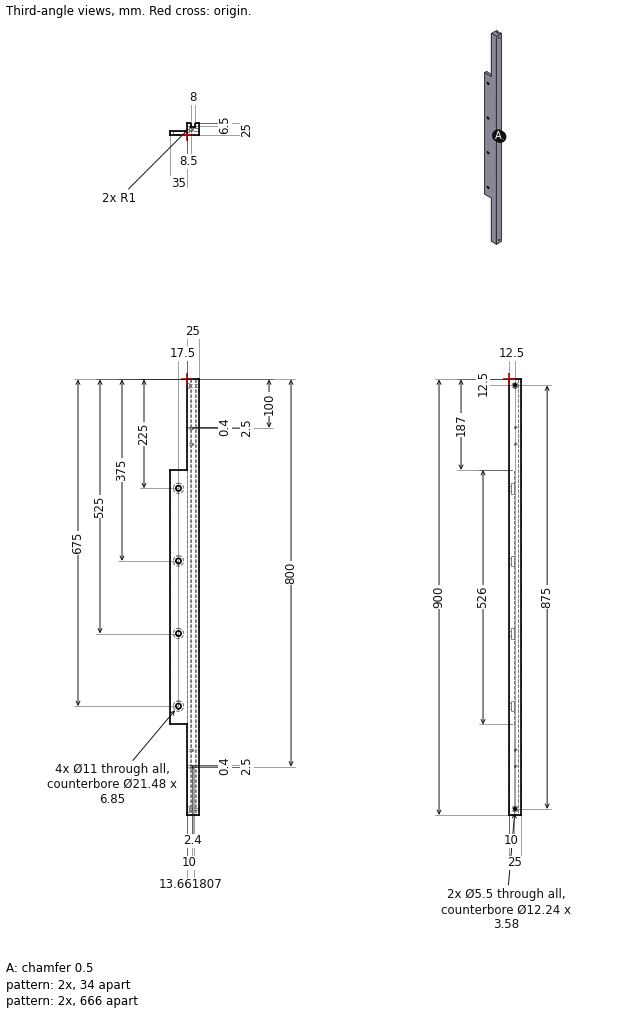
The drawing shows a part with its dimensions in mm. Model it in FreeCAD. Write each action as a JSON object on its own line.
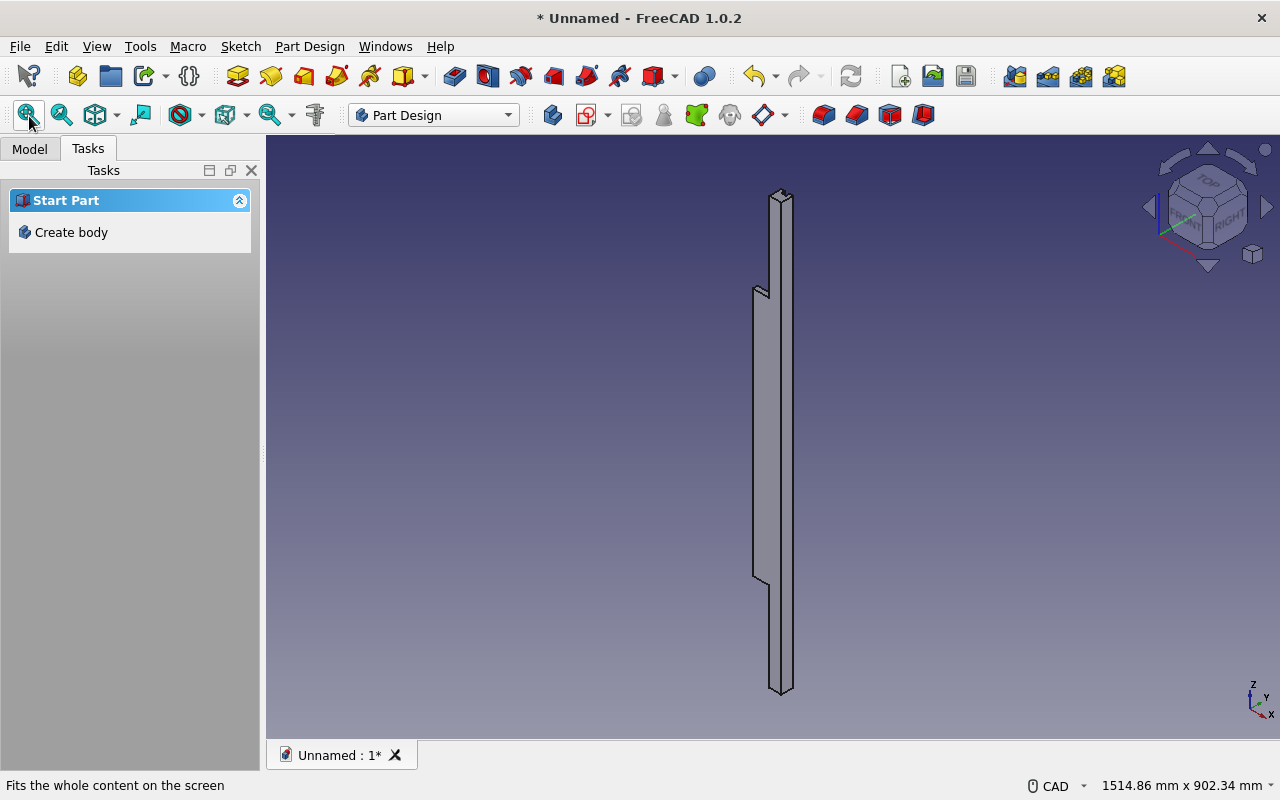
{"action": "key", "text": "2"}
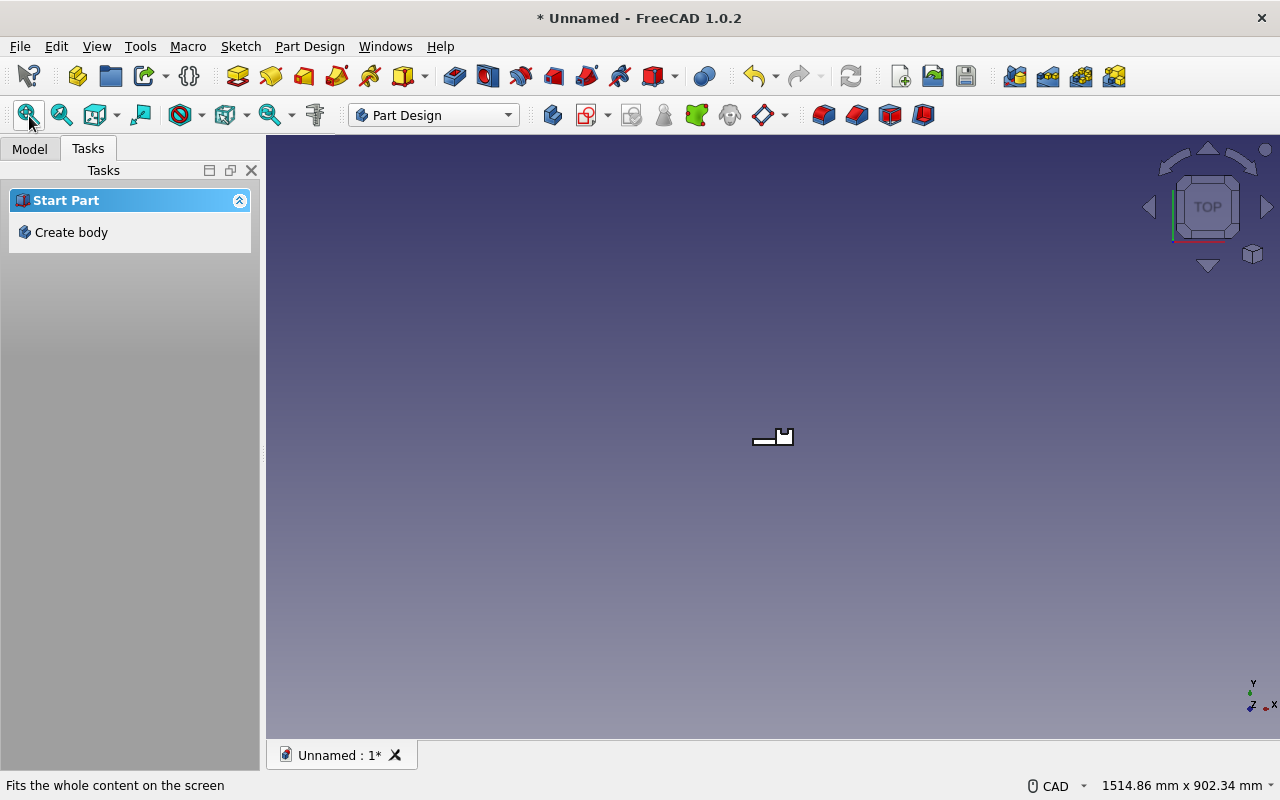
{"action": "left_click", "coordinate": [29, 116]}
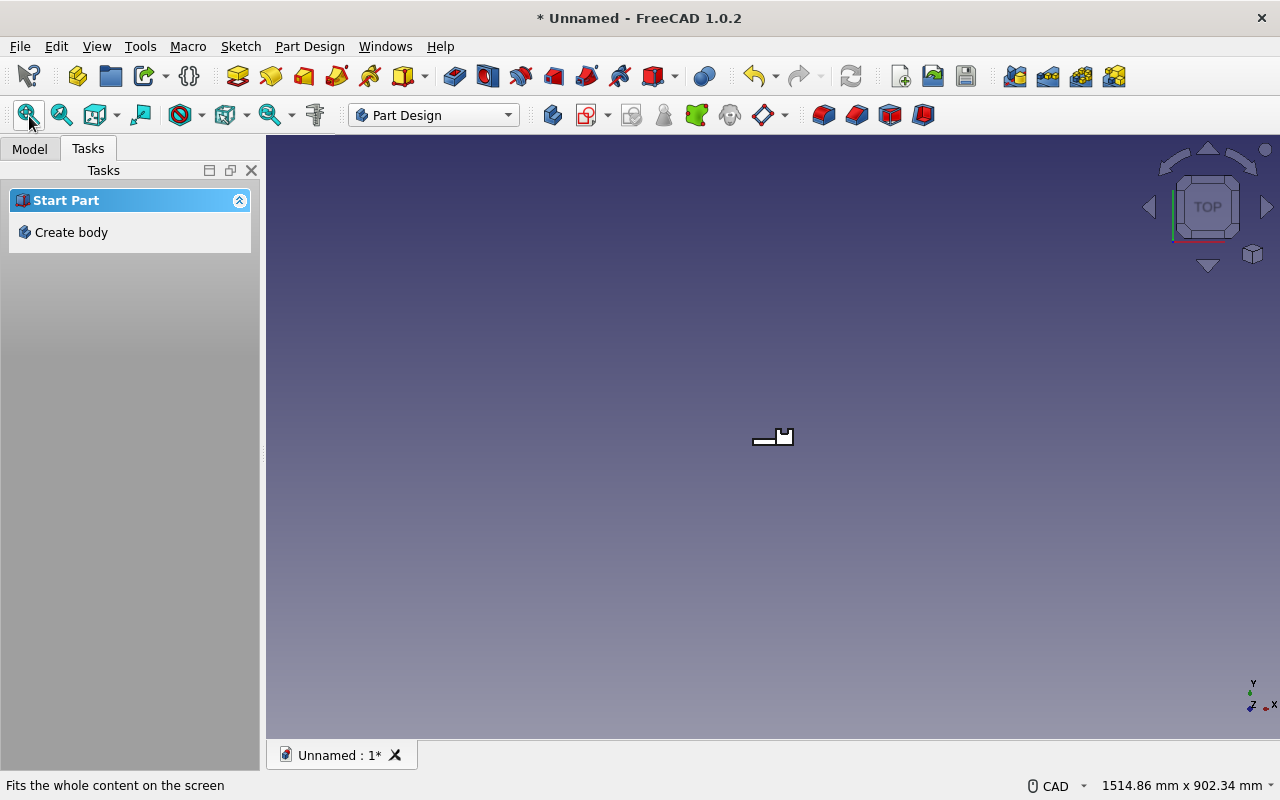
{"action": "key", "text": "1"}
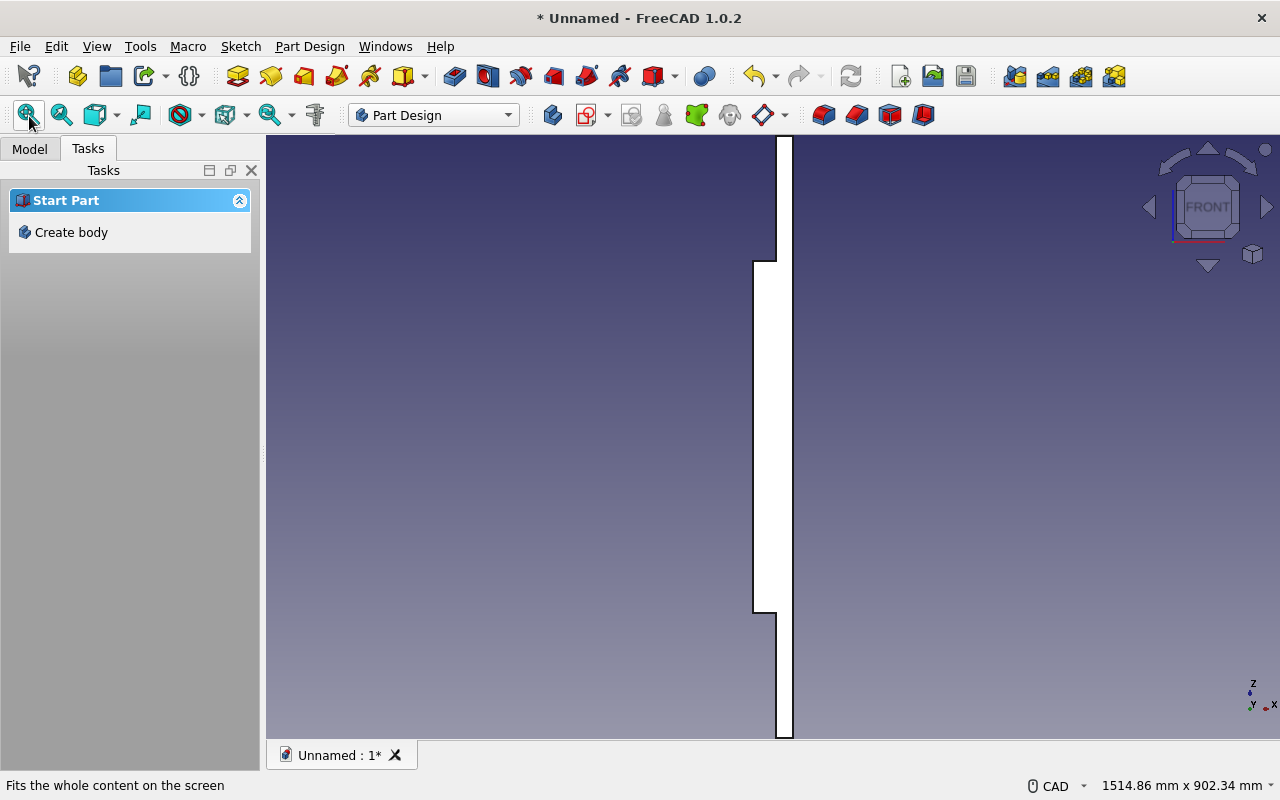
{"action": "key", "text": "3"}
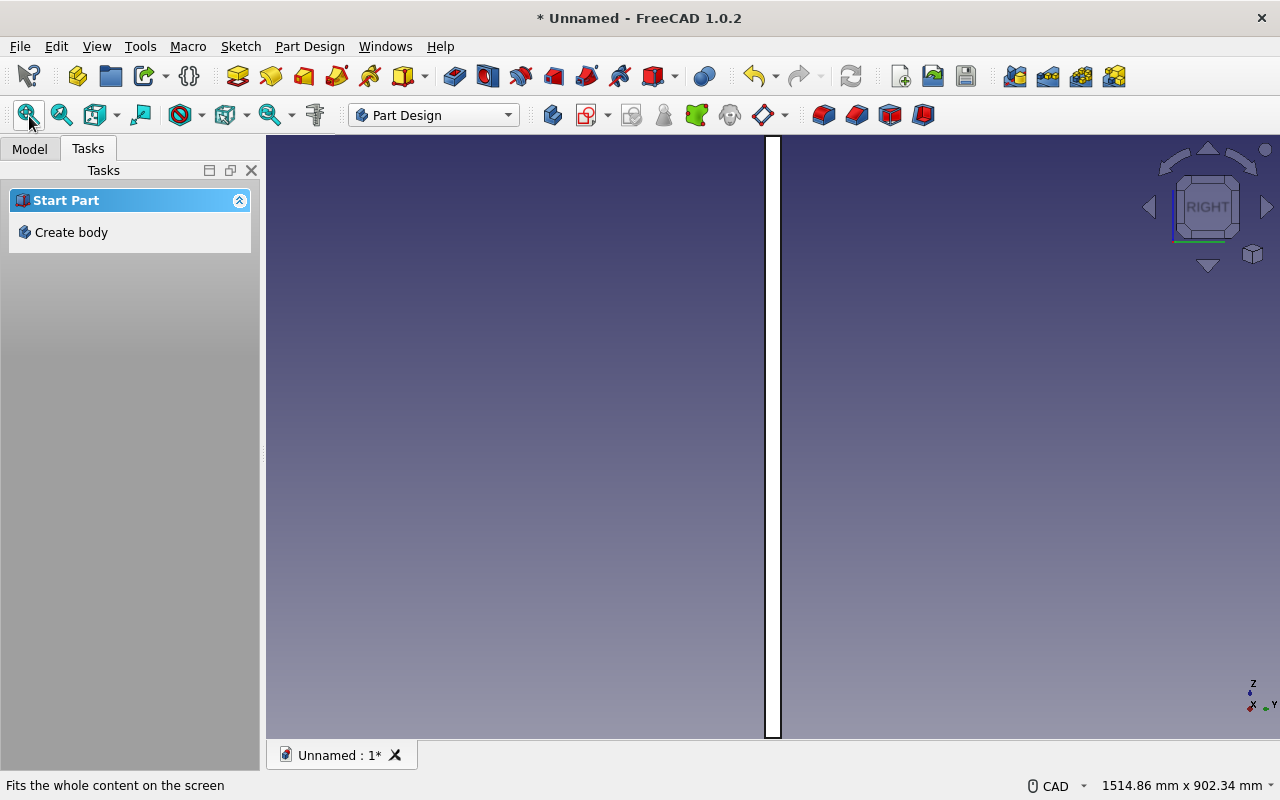
{"action": "key", "text": "5"}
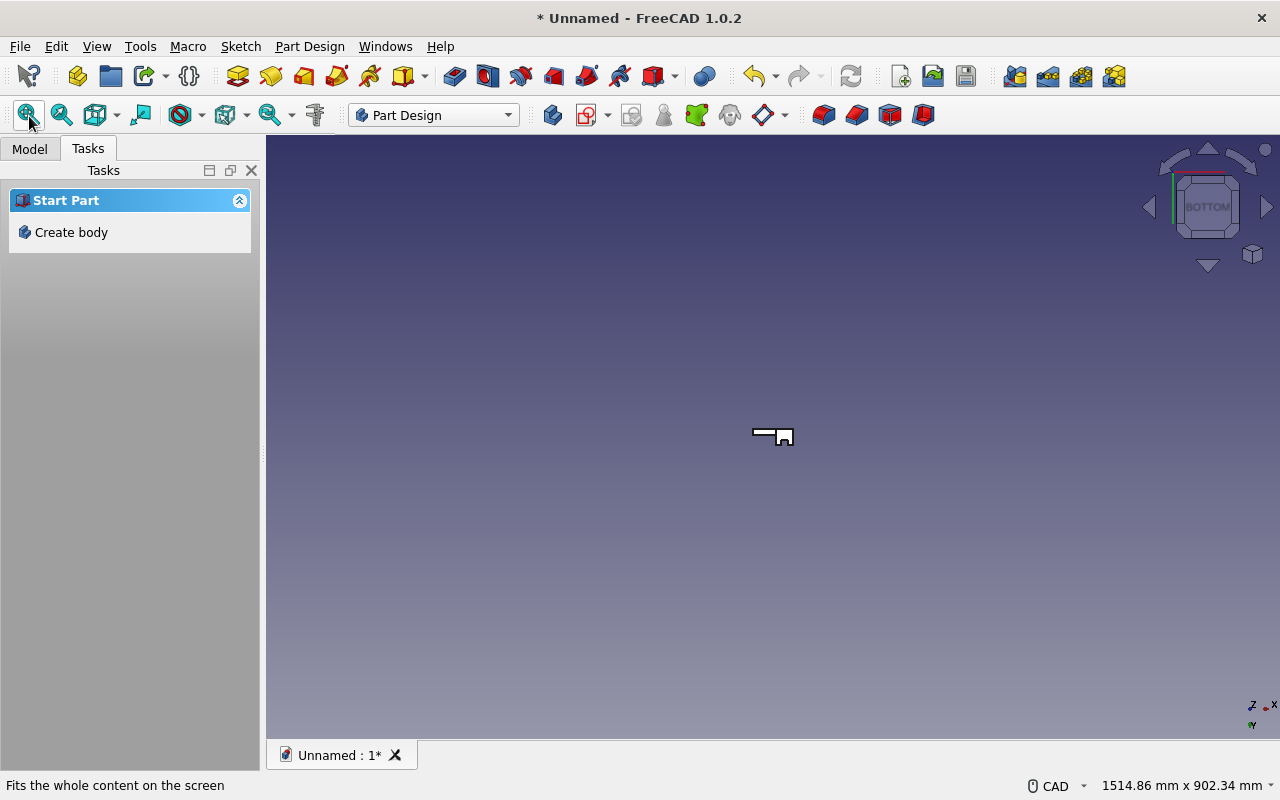
{"action": "left_click", "coordinate": [29, 116]}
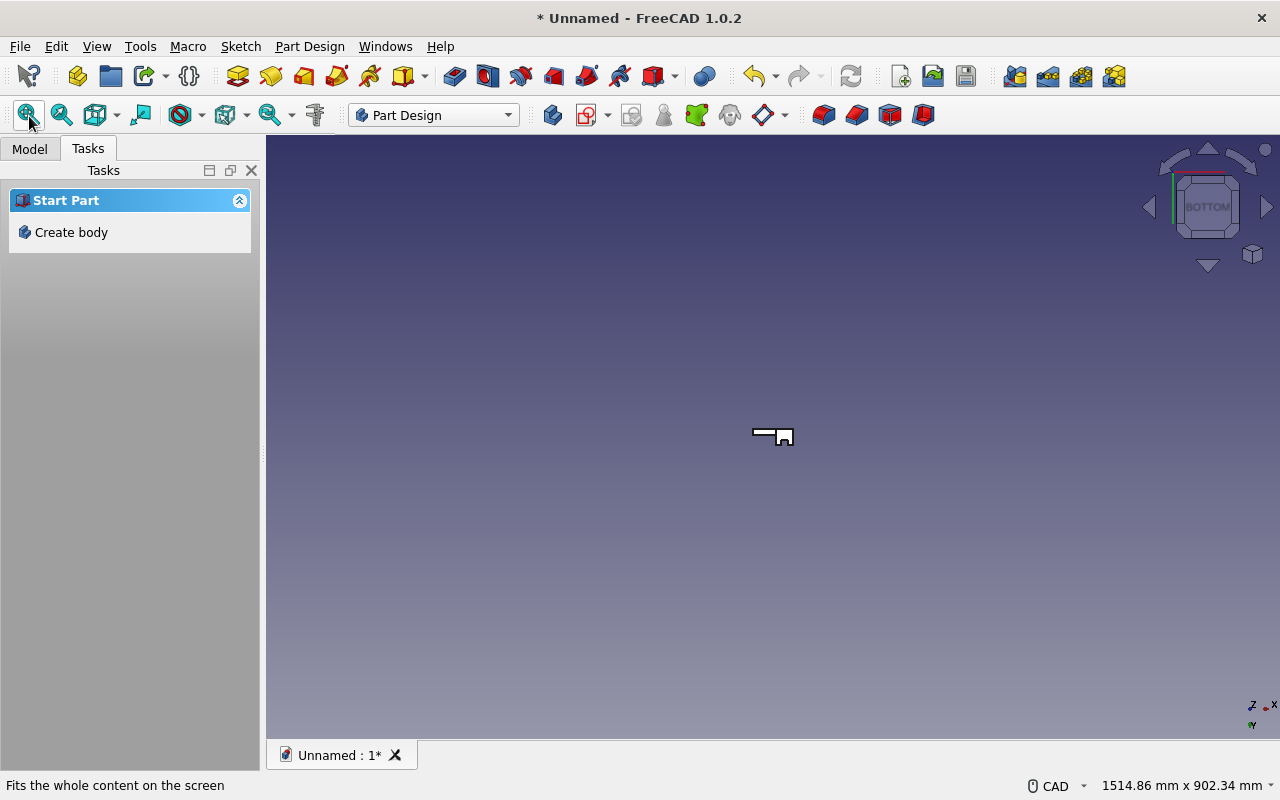
{"action": "key", "text": "4"}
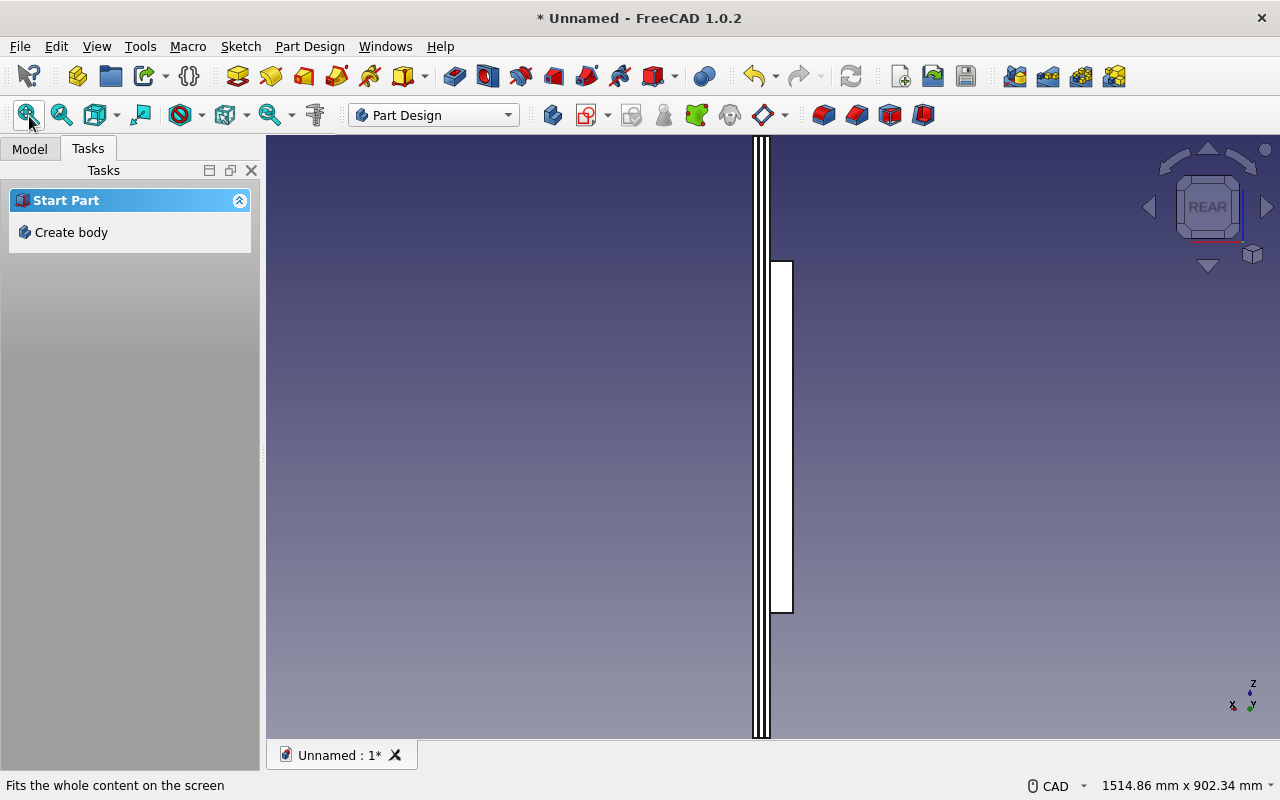
{"action": "key", "text": "6"}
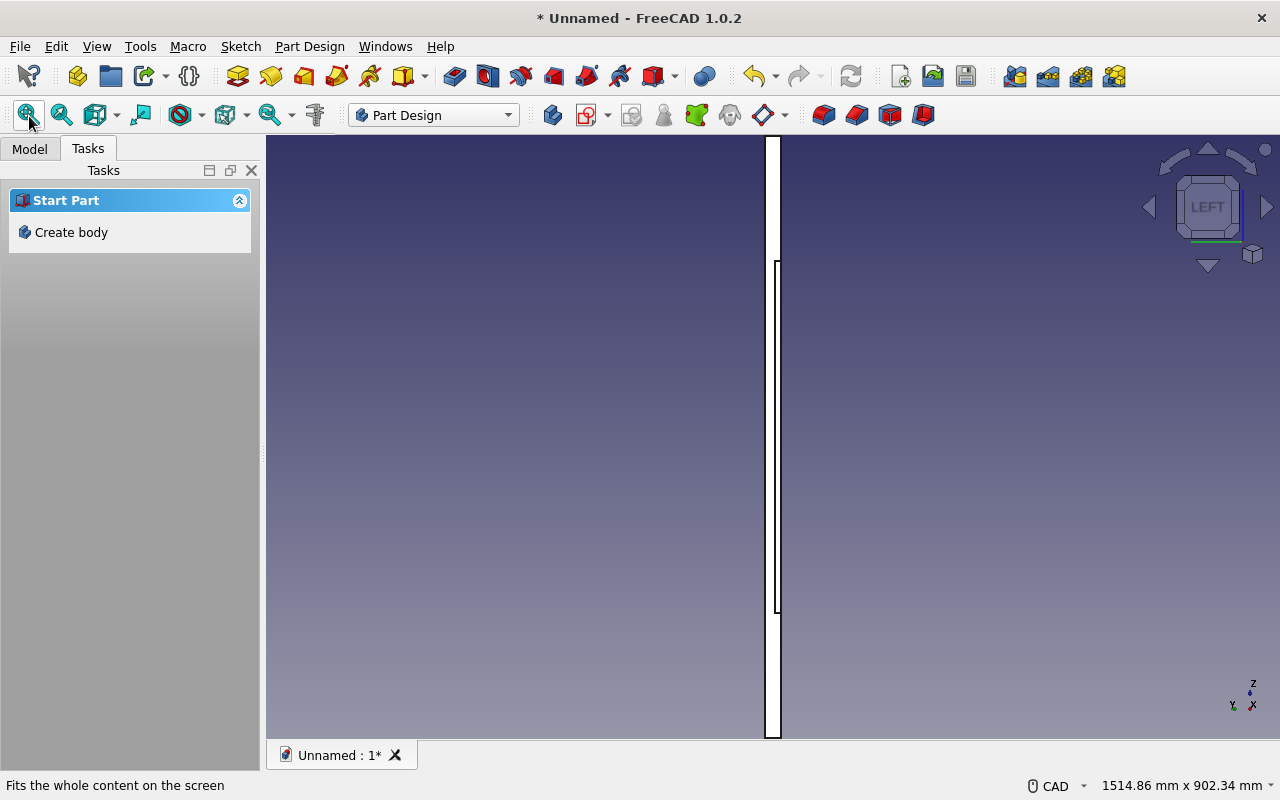
{"action": "key", "text": "v 3"}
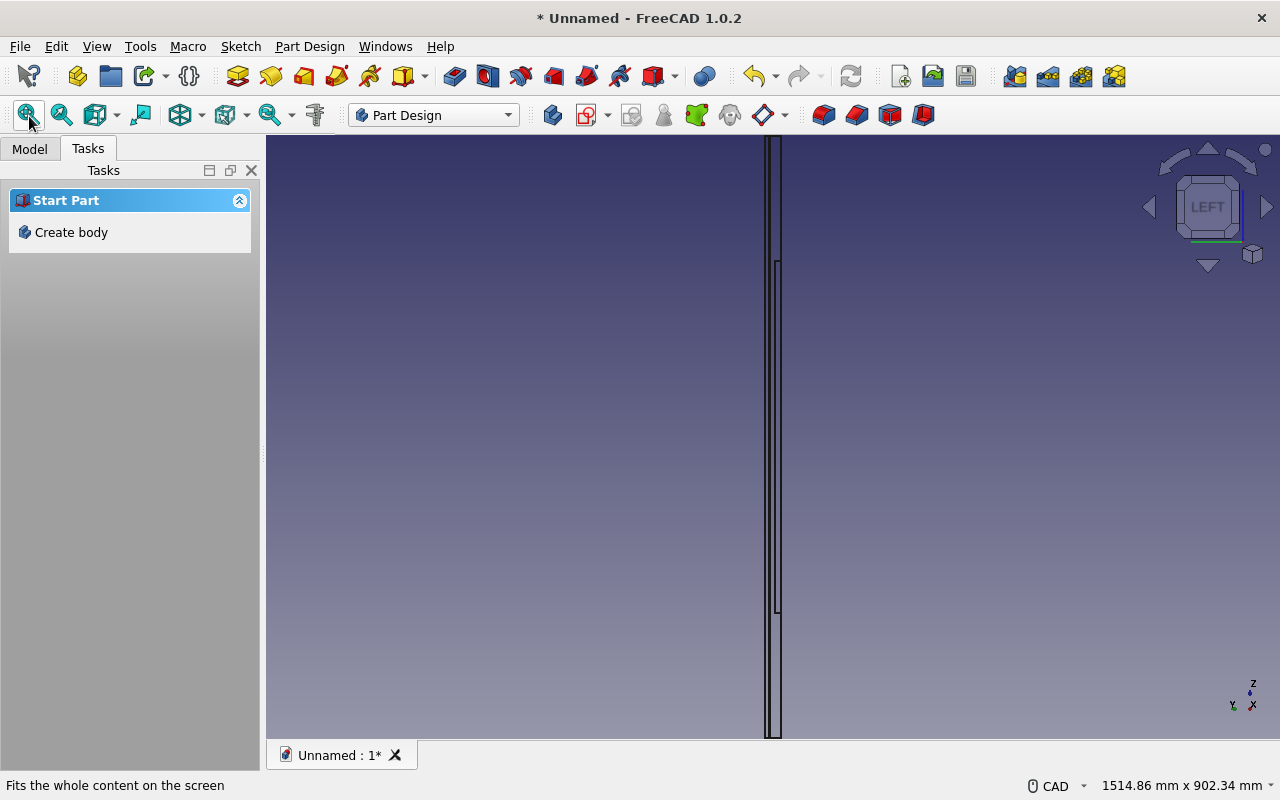
{"action": "key", "text": "0"}